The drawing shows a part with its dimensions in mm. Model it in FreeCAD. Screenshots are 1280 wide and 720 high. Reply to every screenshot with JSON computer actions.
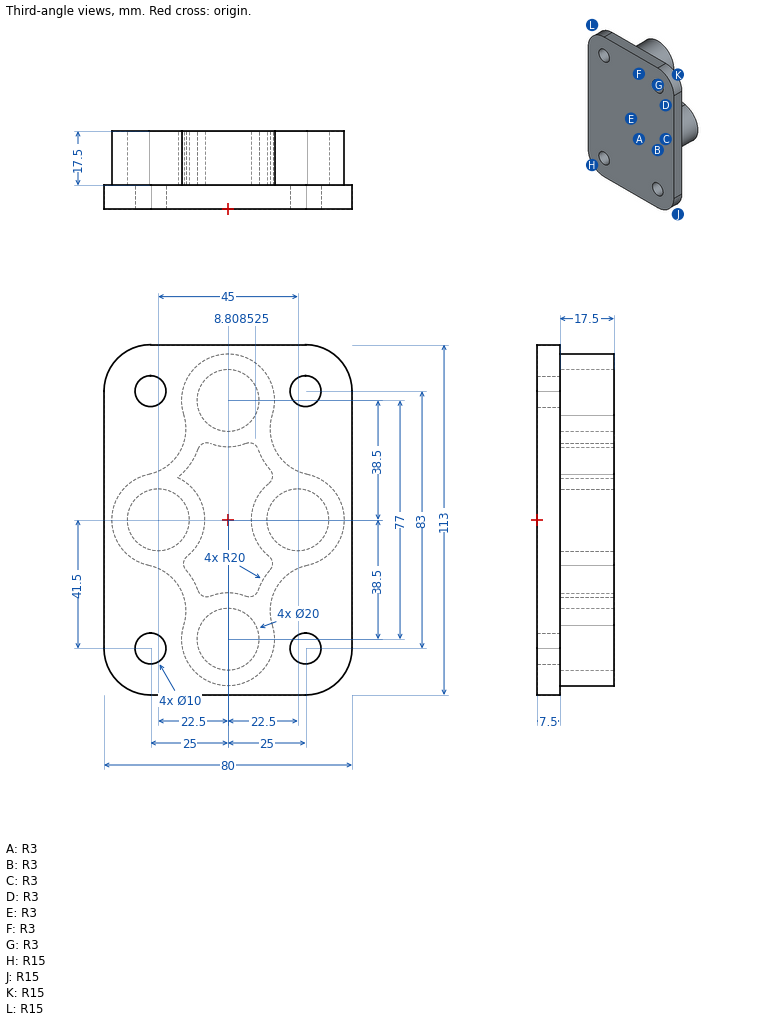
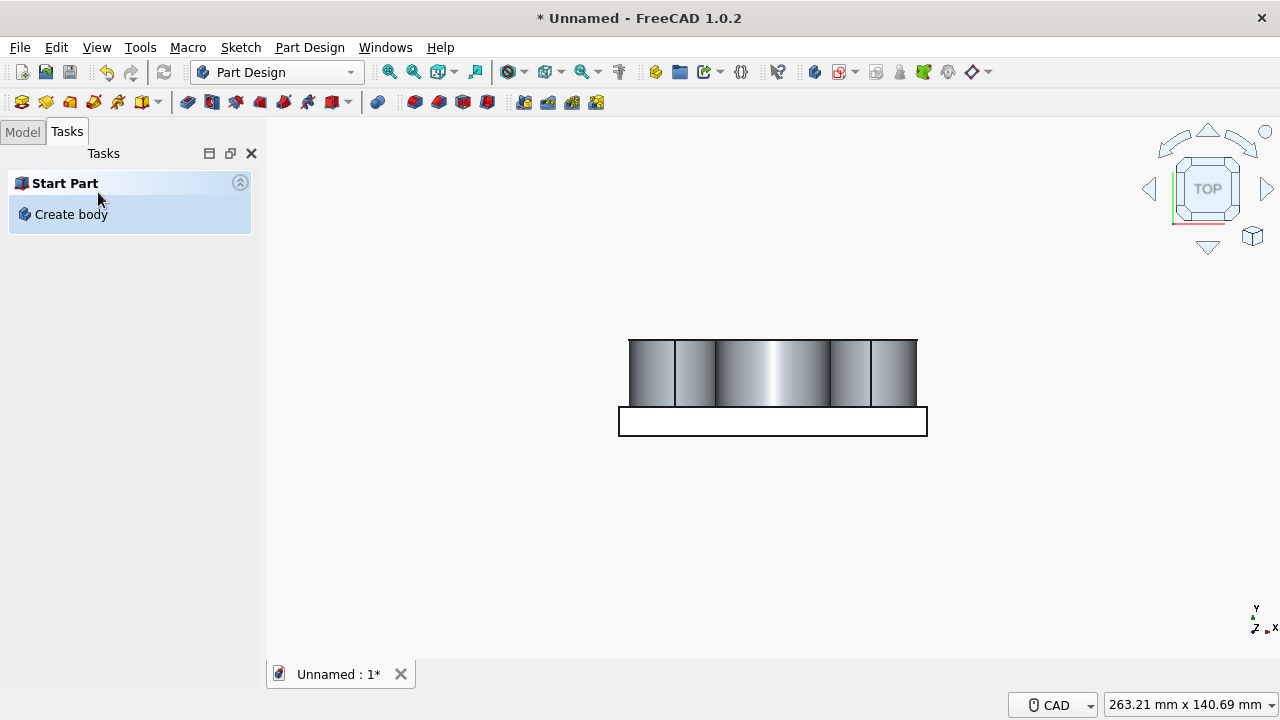
{"action": "key", "text": "0"}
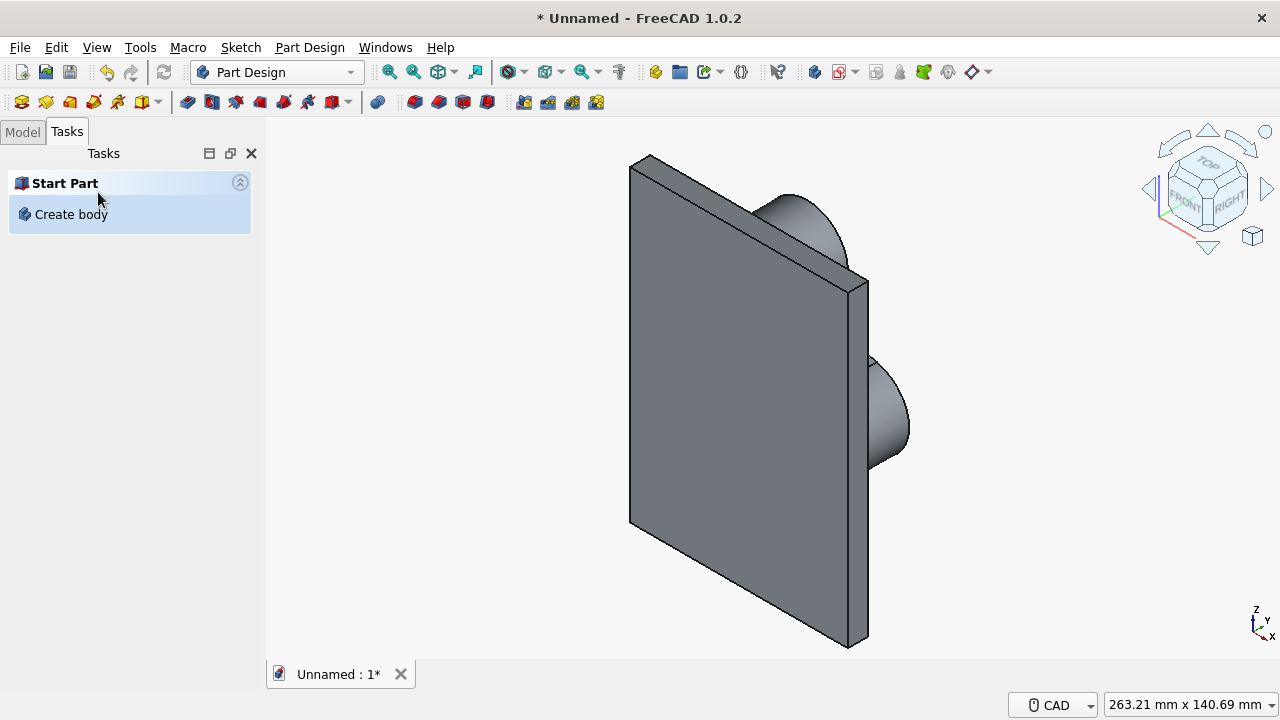
{"action": "key", "text": "1"}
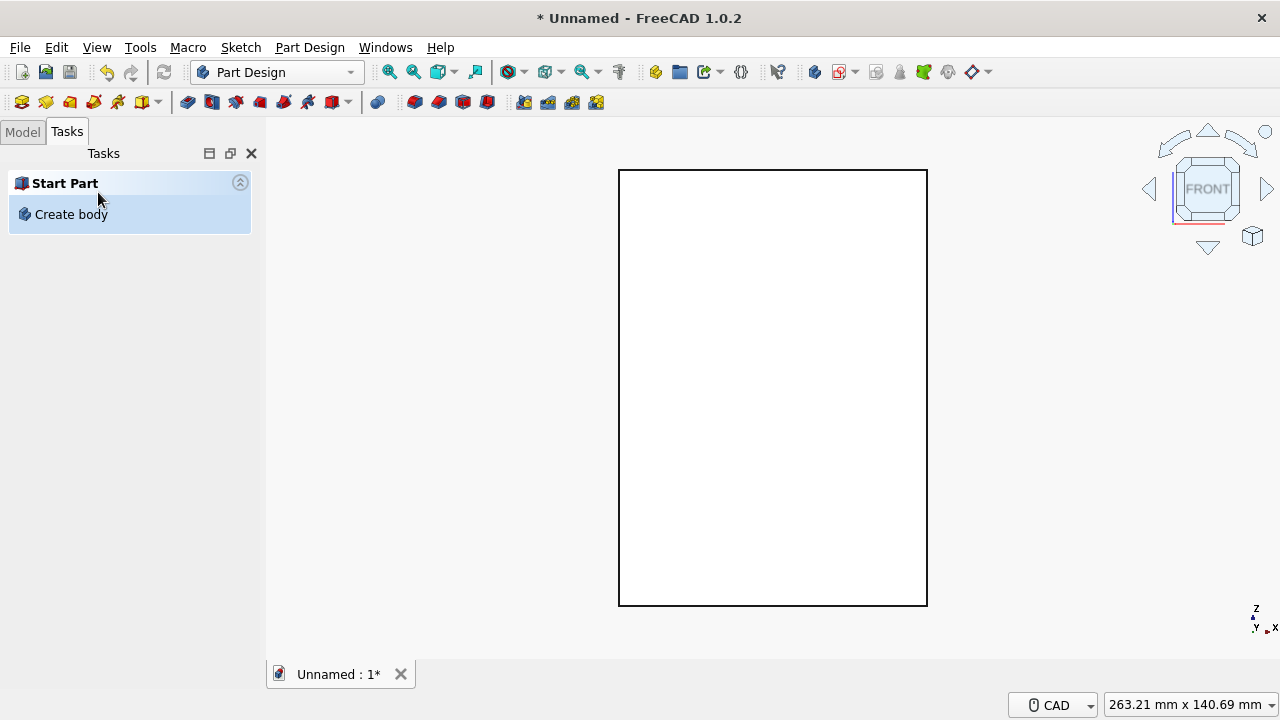
{"action": "key", "text": "3"}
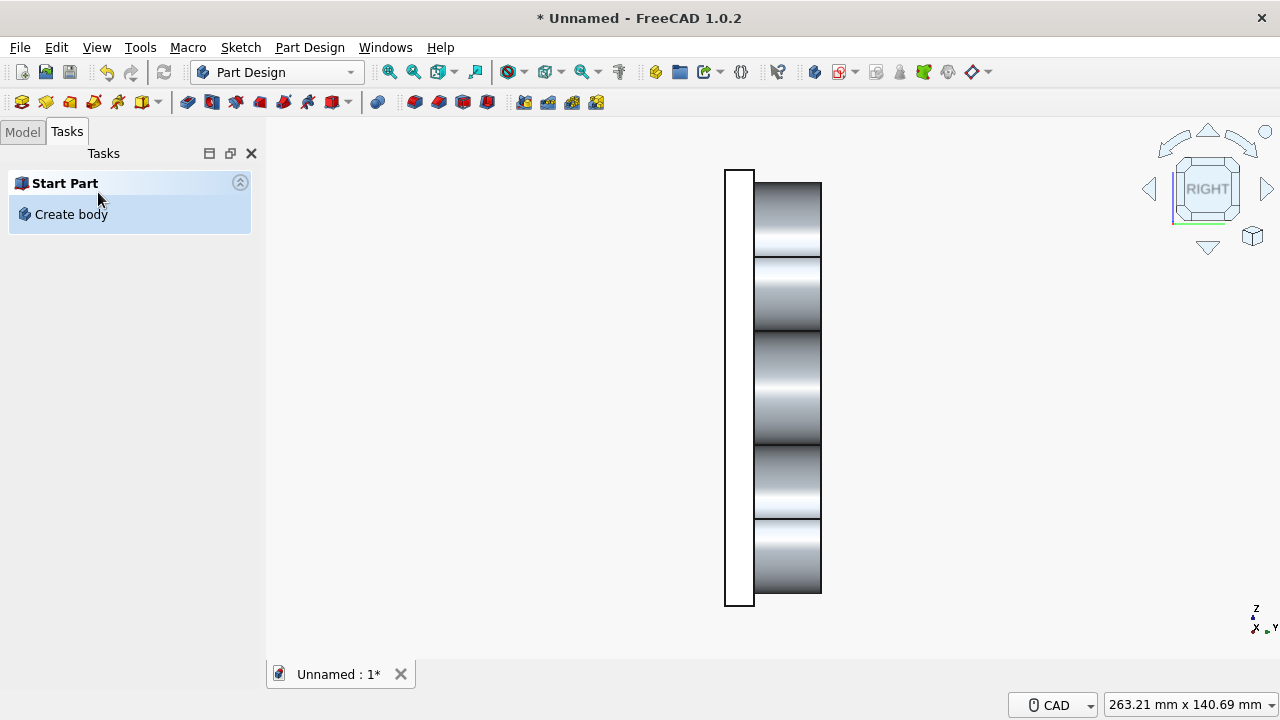
{"action": "key", "text": "5"}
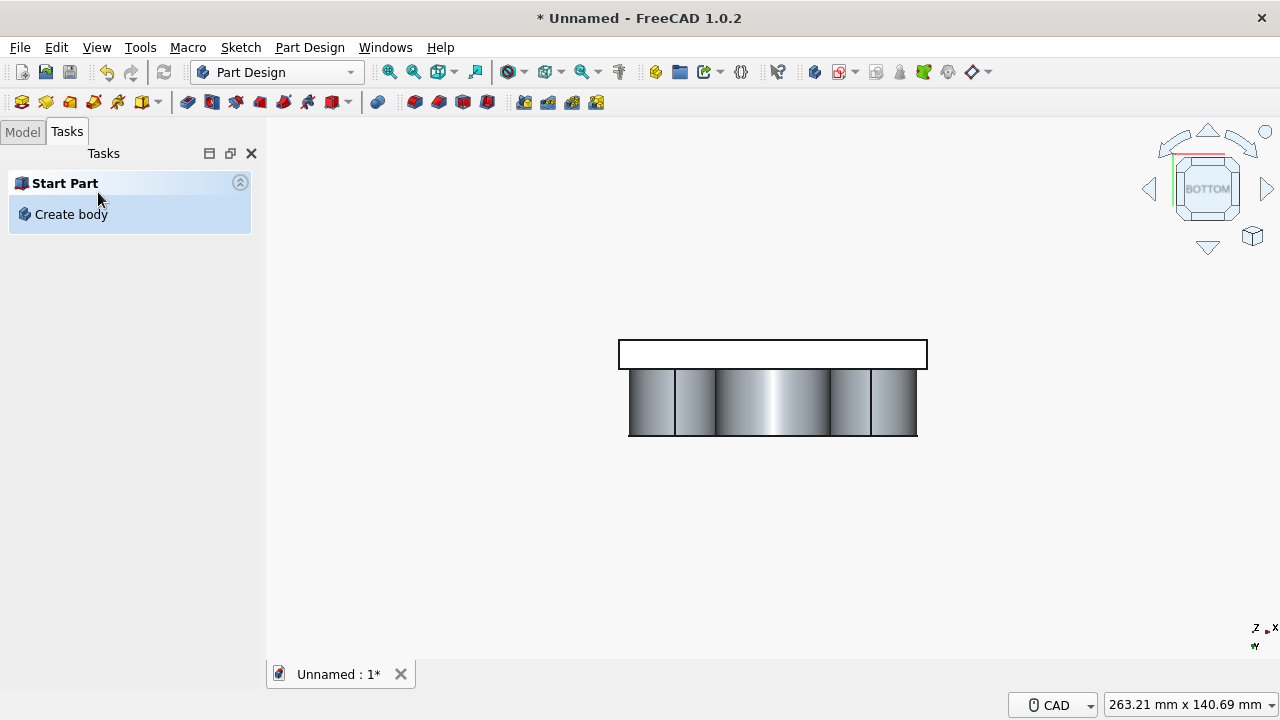
{"action": "key", "text": "v f"}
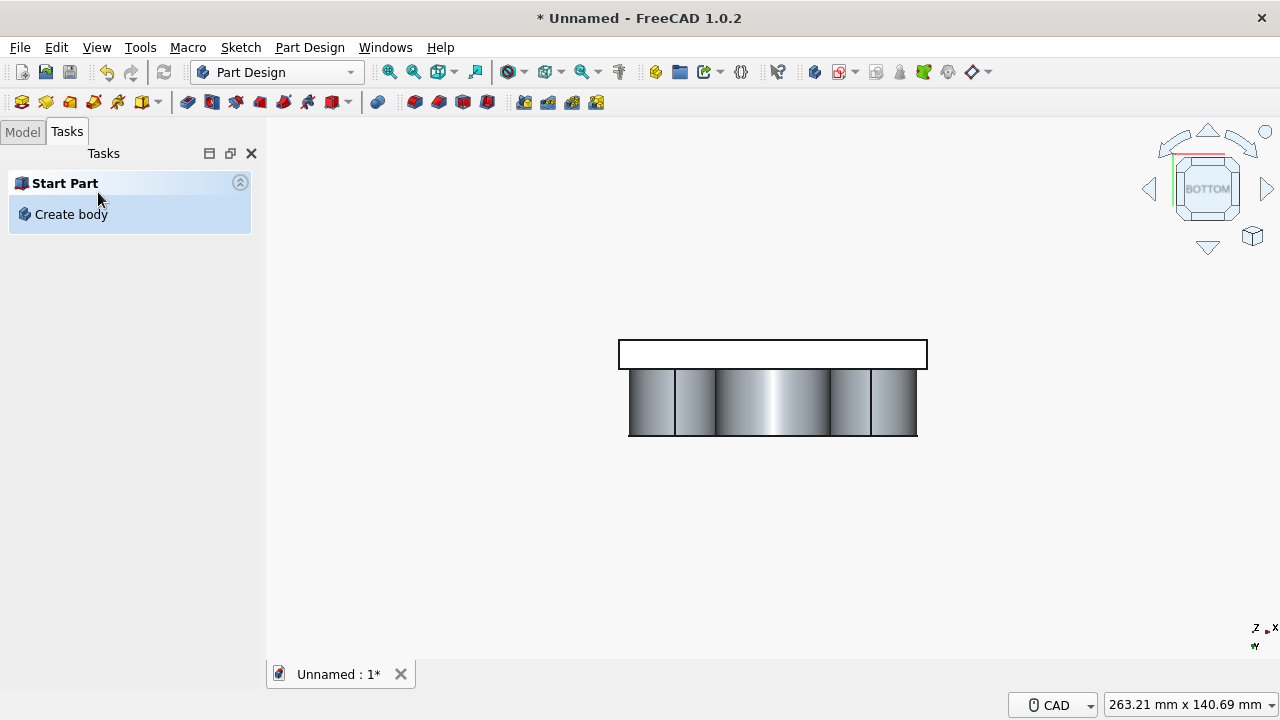
{"action": "key", "text": "4"}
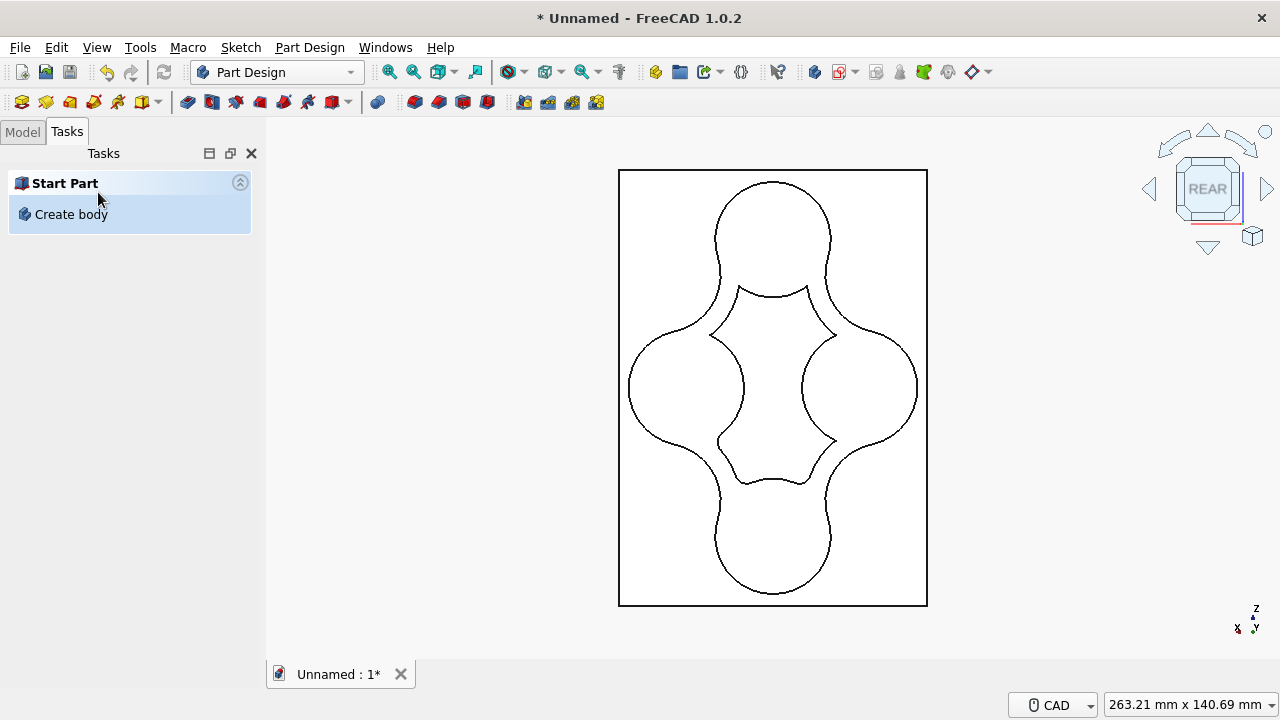
{"action": "key", "text": "6"}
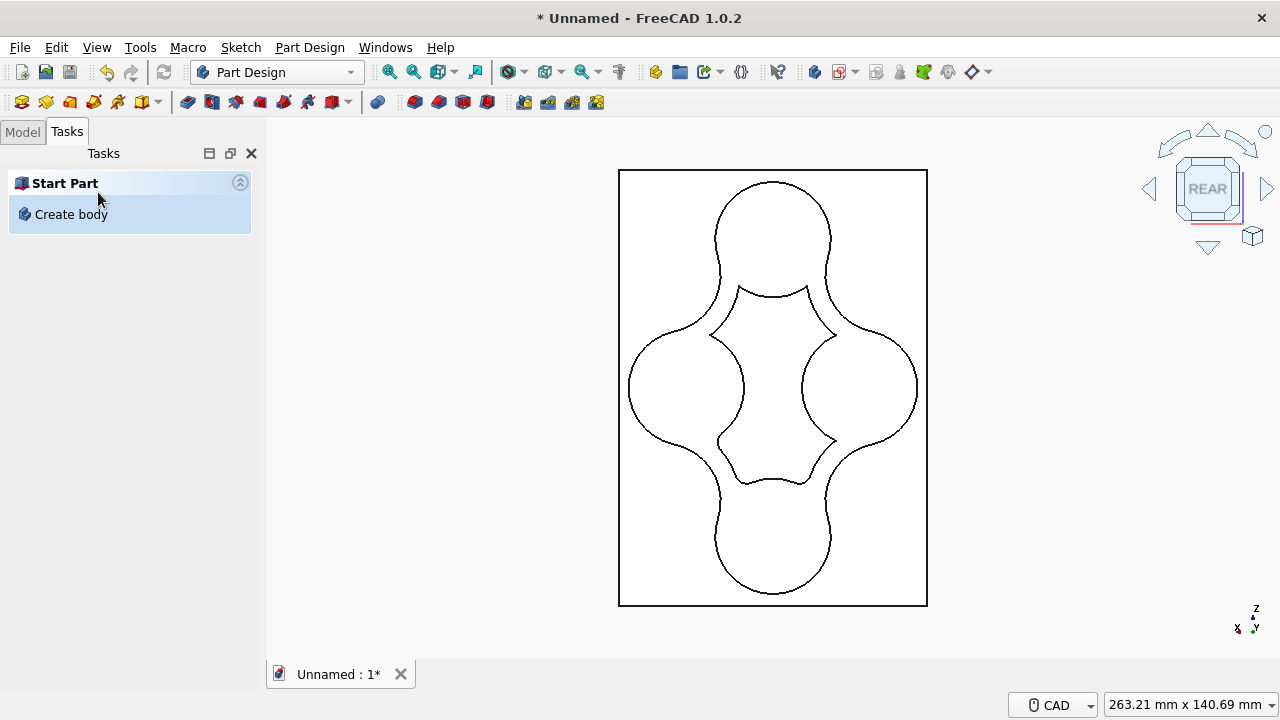
{"action": "key", "text": "v 3"}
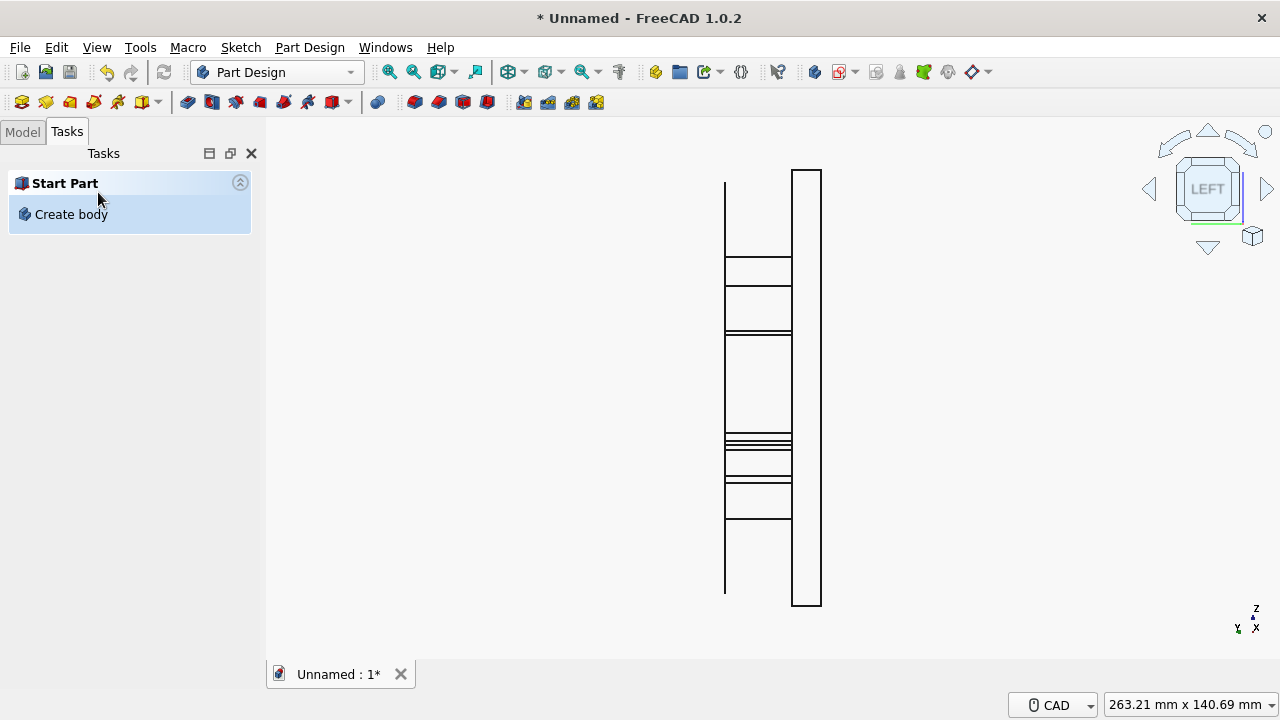
{"action": "key", "text": "0"}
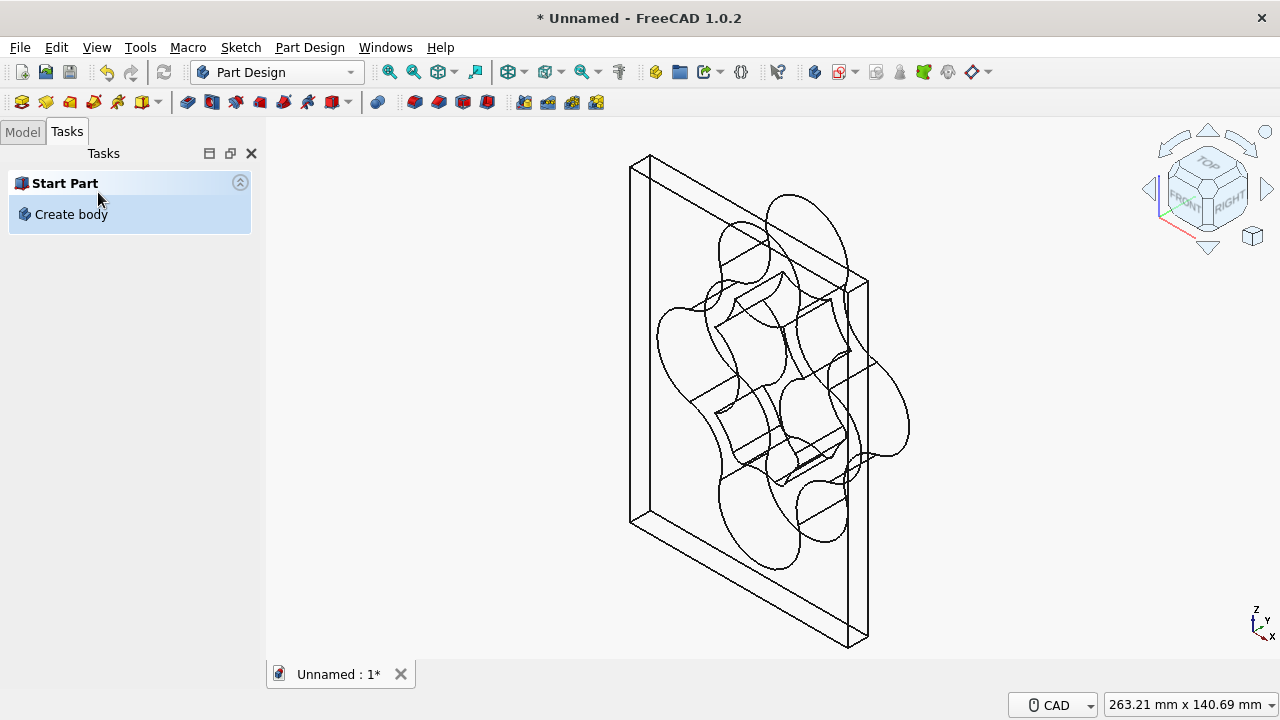
{"action": "left_click", "coordinate": [827, 364]}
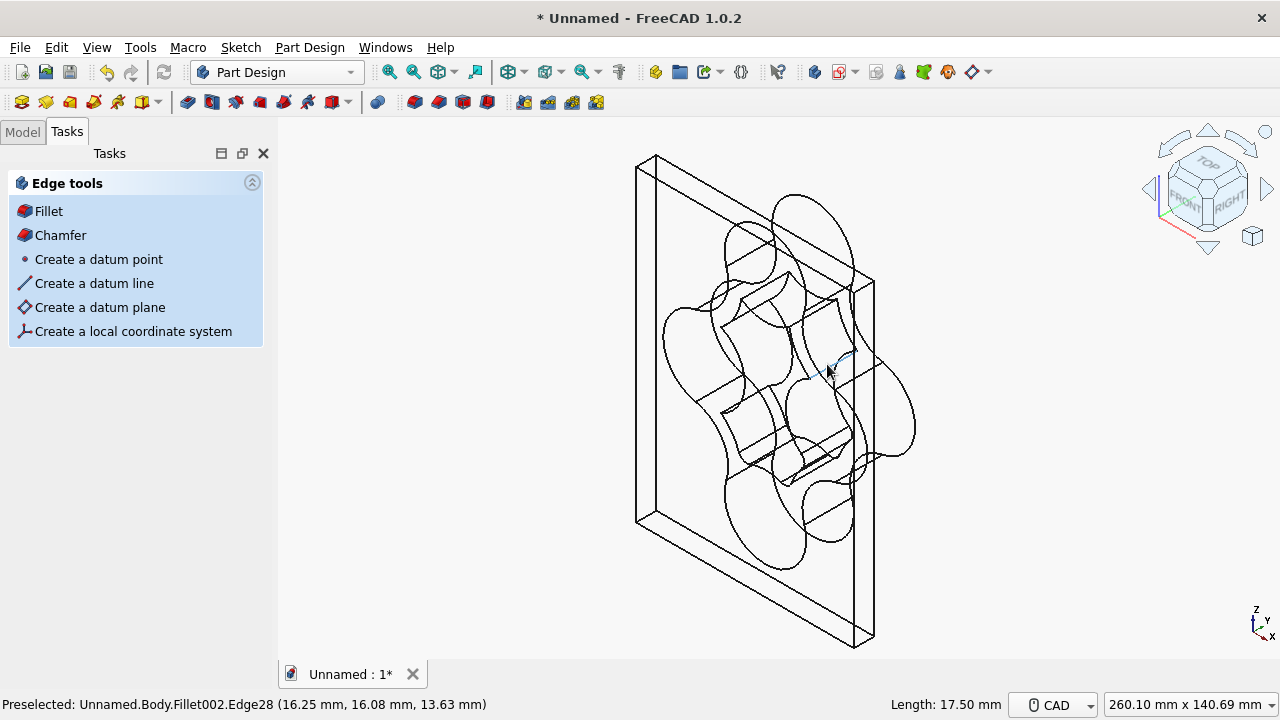
{"action": "key", "text": "v 1"}